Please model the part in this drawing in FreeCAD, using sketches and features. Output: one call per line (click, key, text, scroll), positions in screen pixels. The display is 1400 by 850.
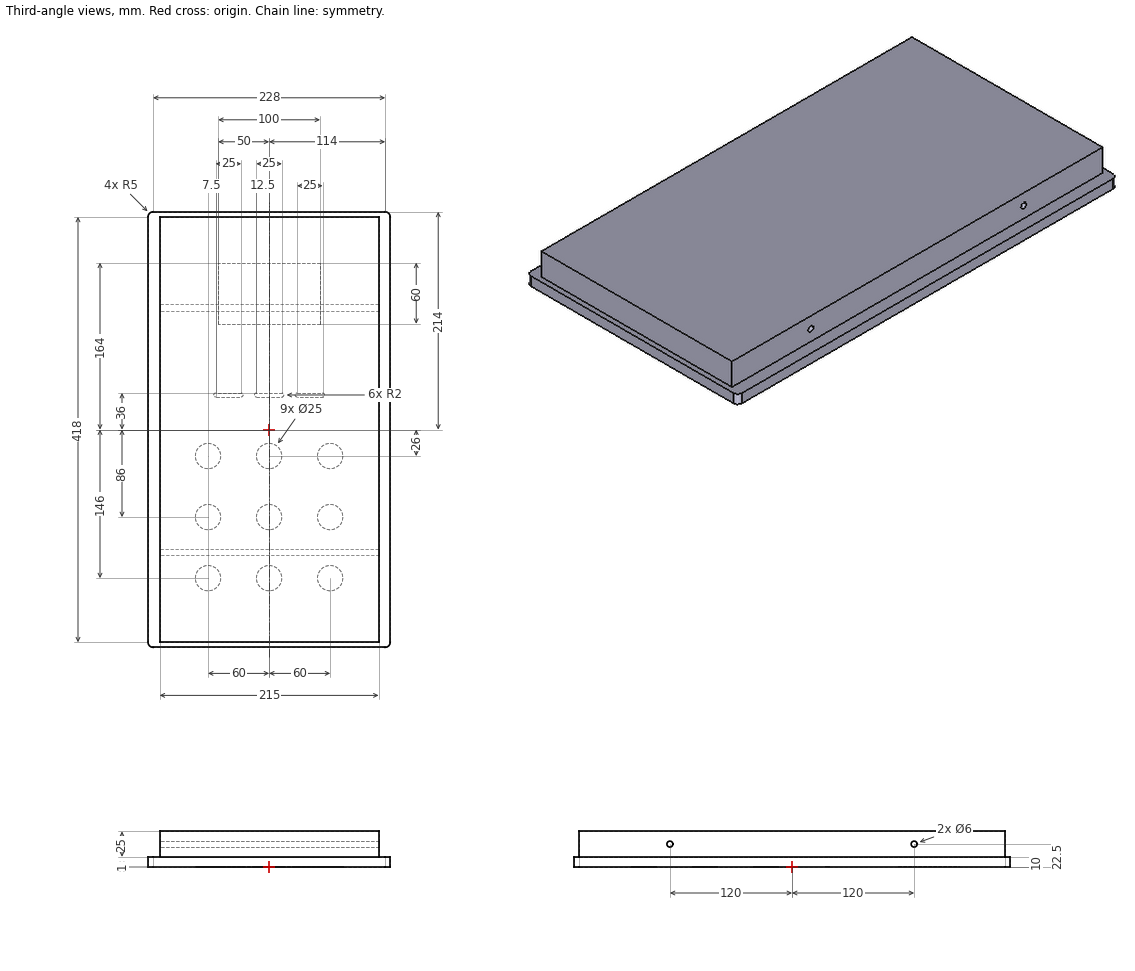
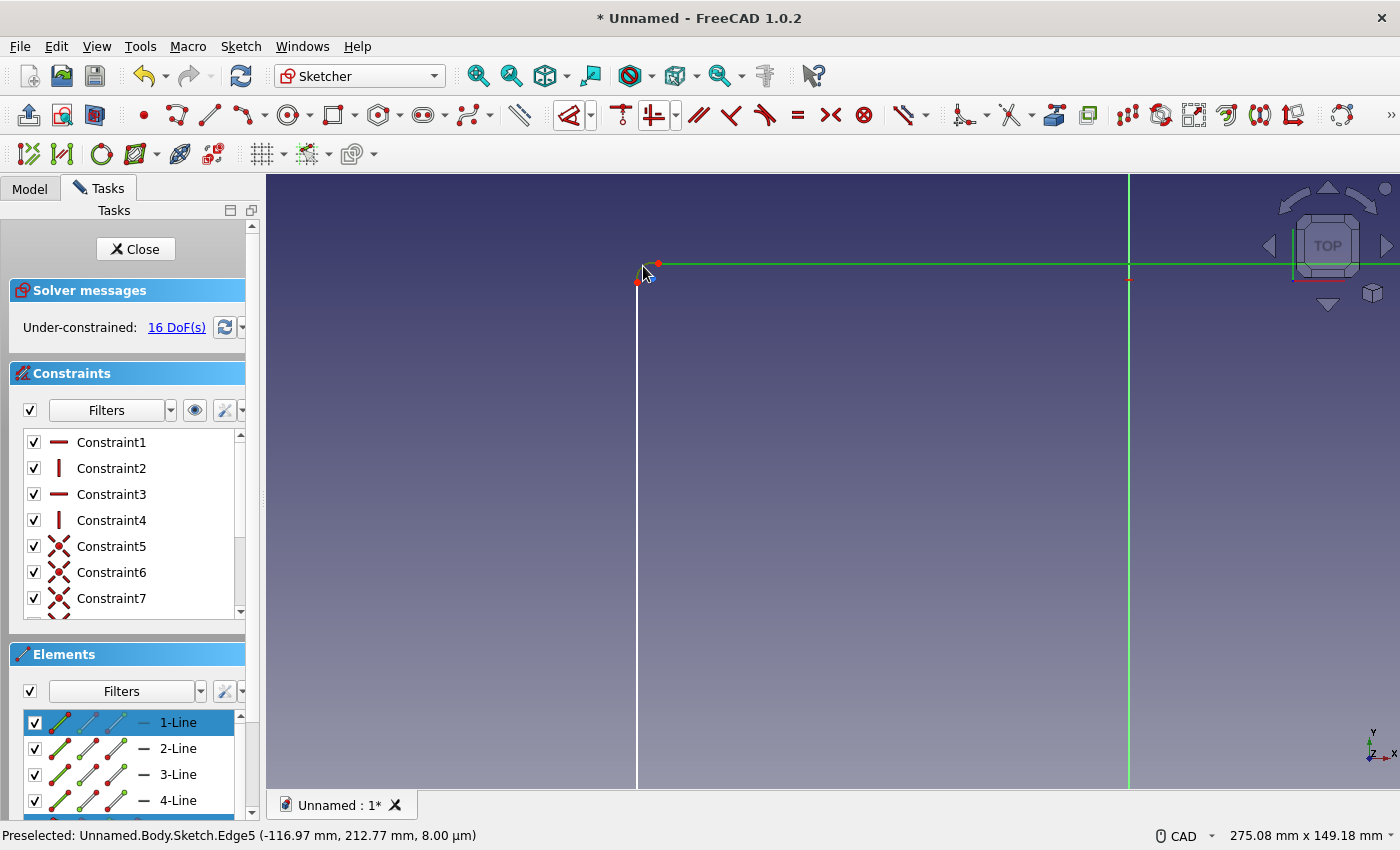
key(t)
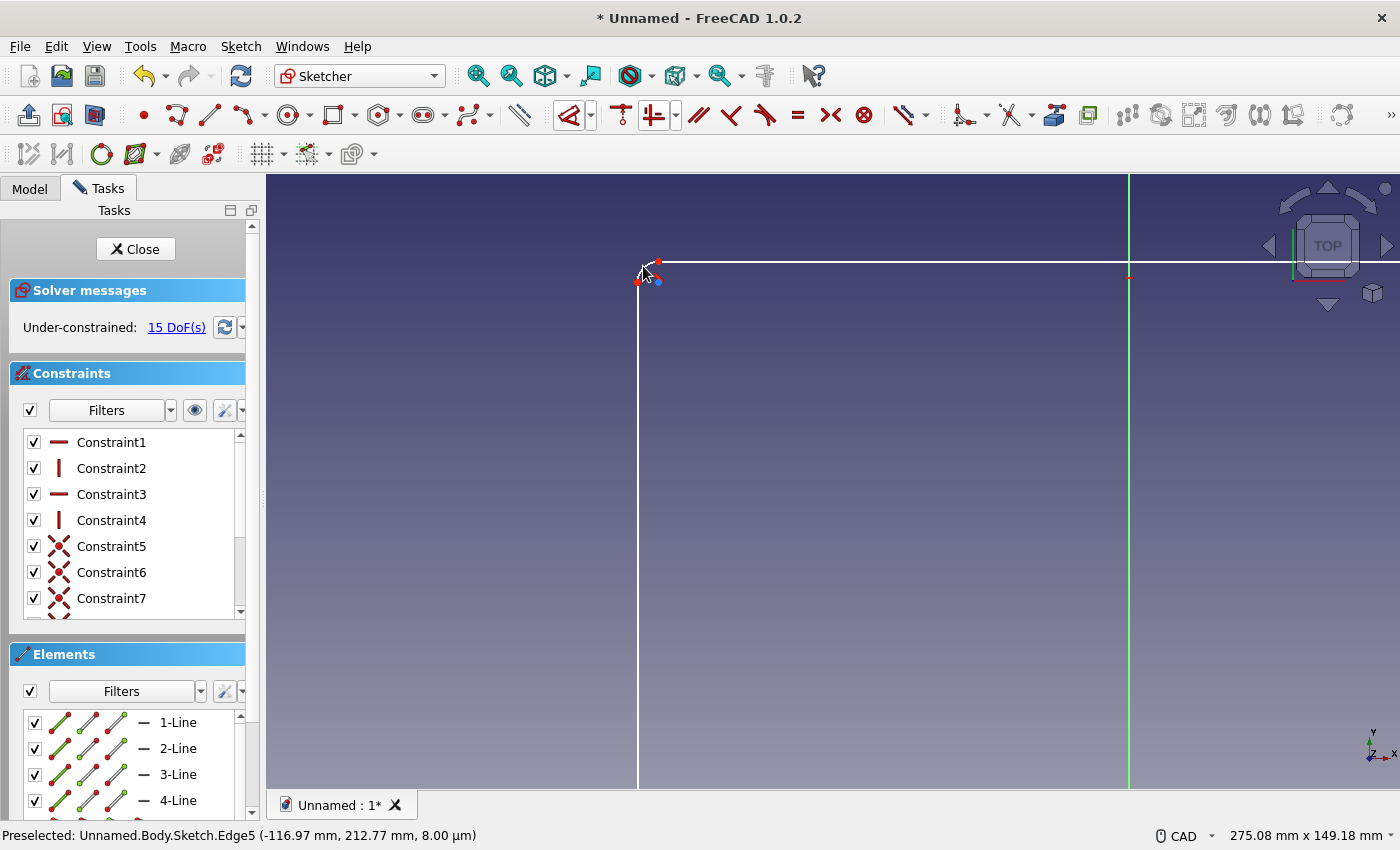
scroll(645, 266, down, 7)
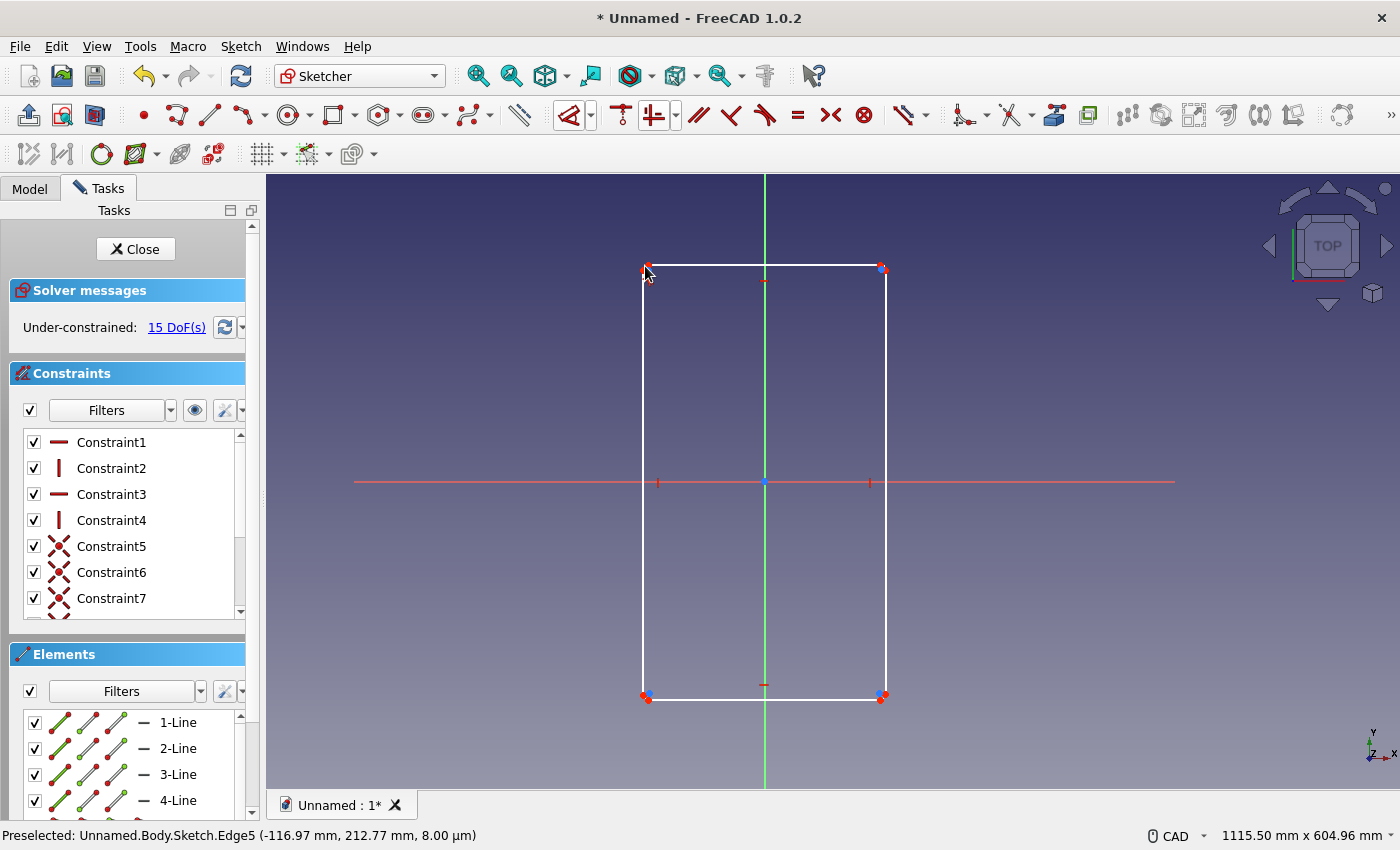
click(718, 265)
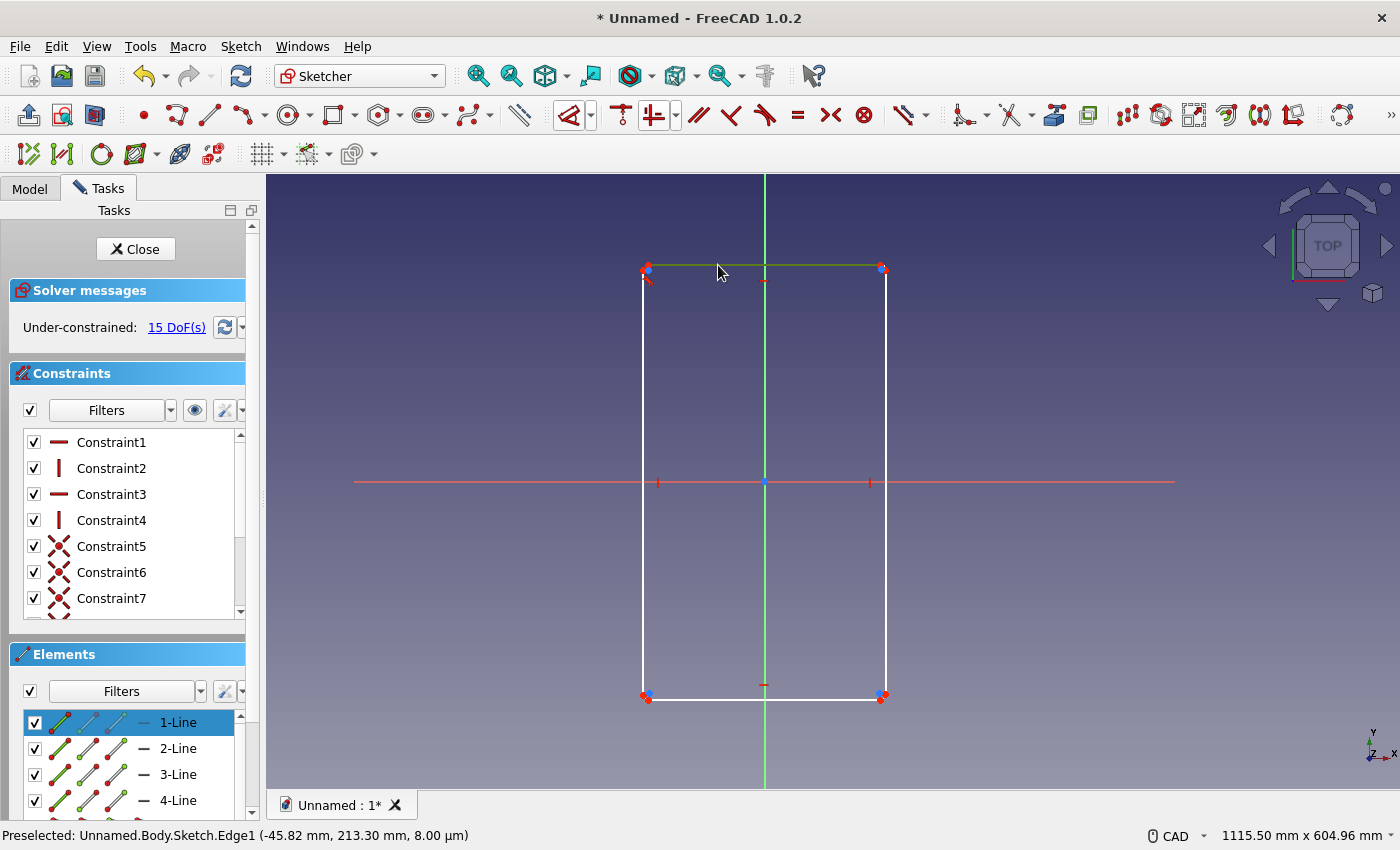
scroll(885, 266, up, 7)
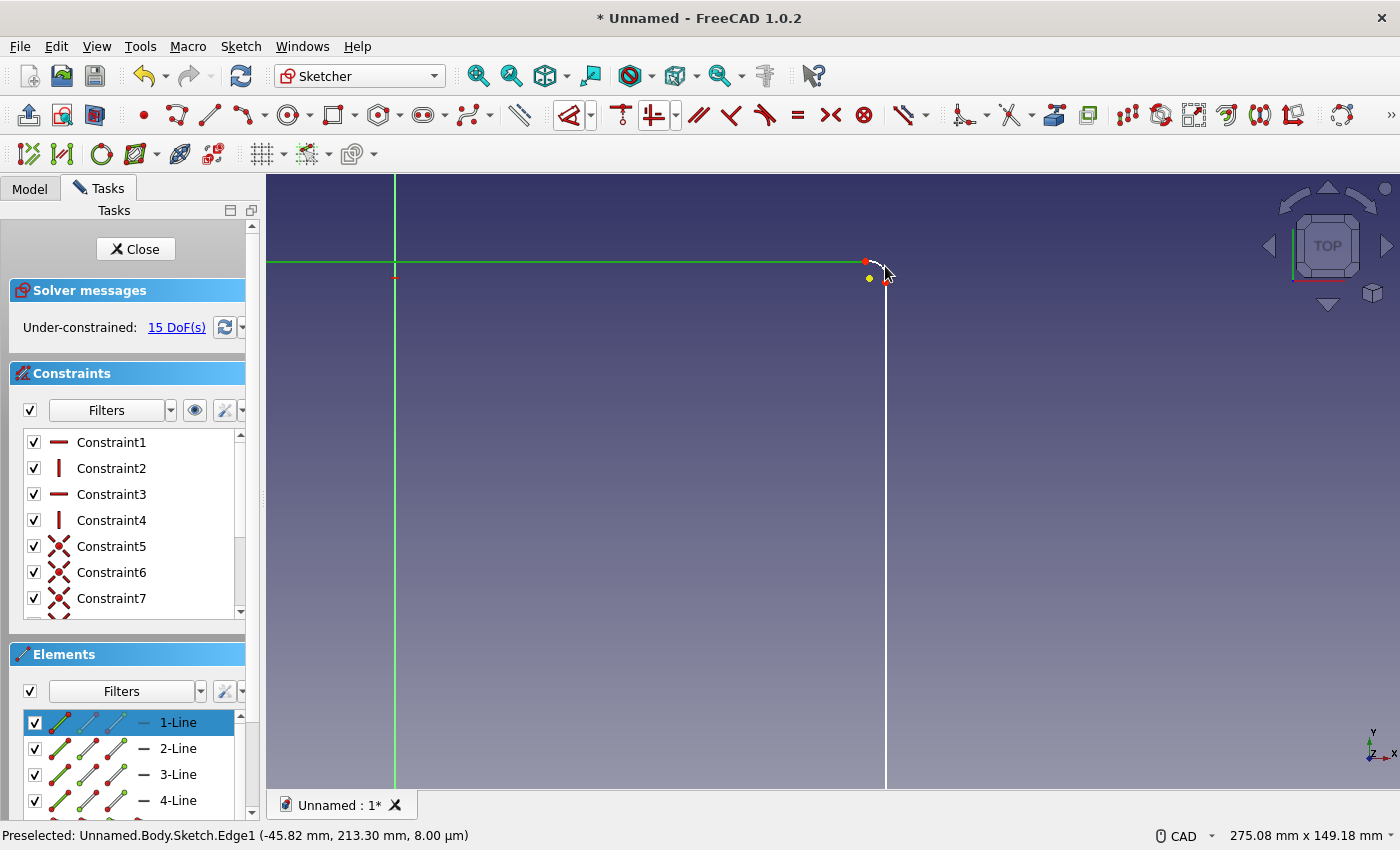
click(882, 266)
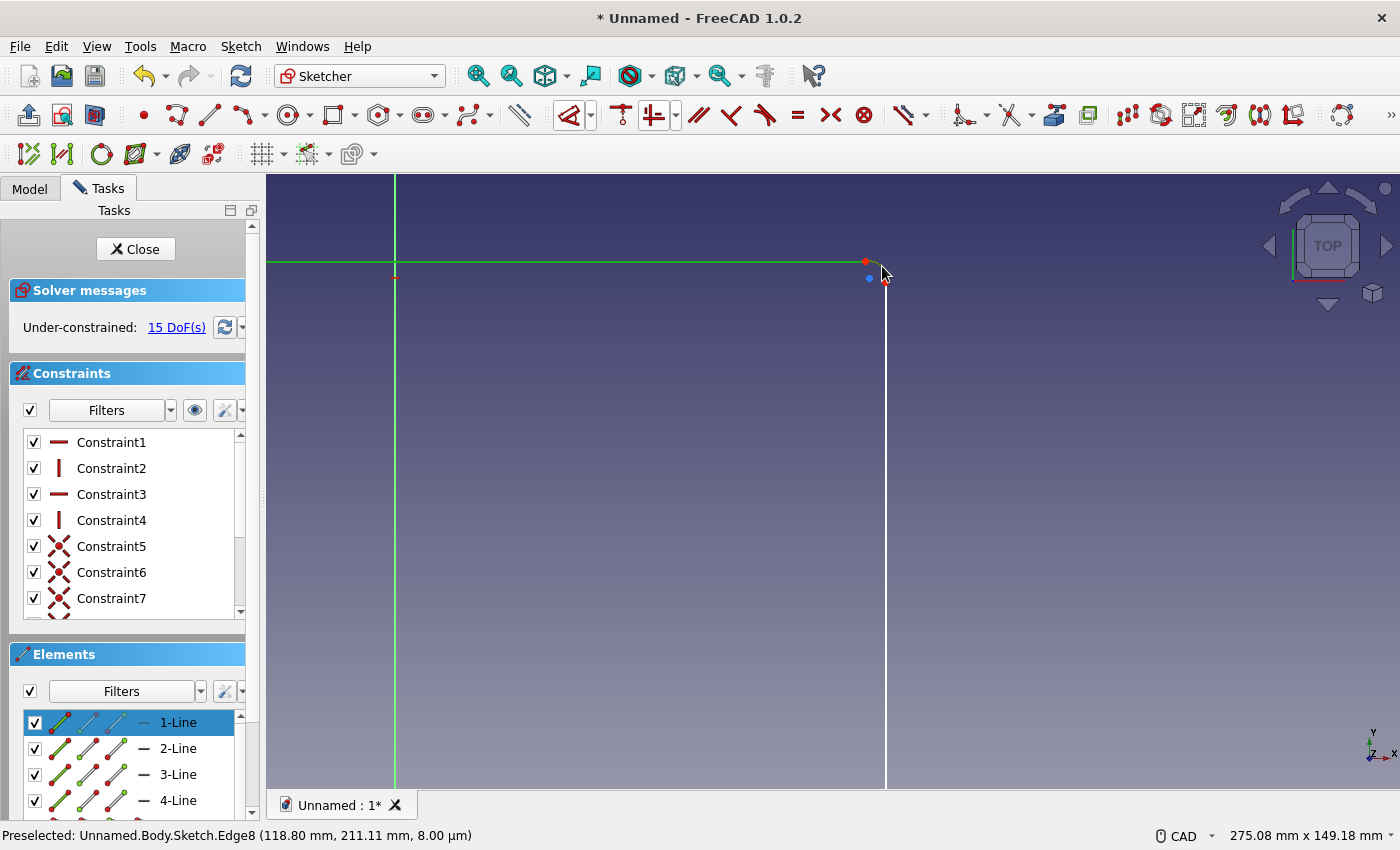
key(t)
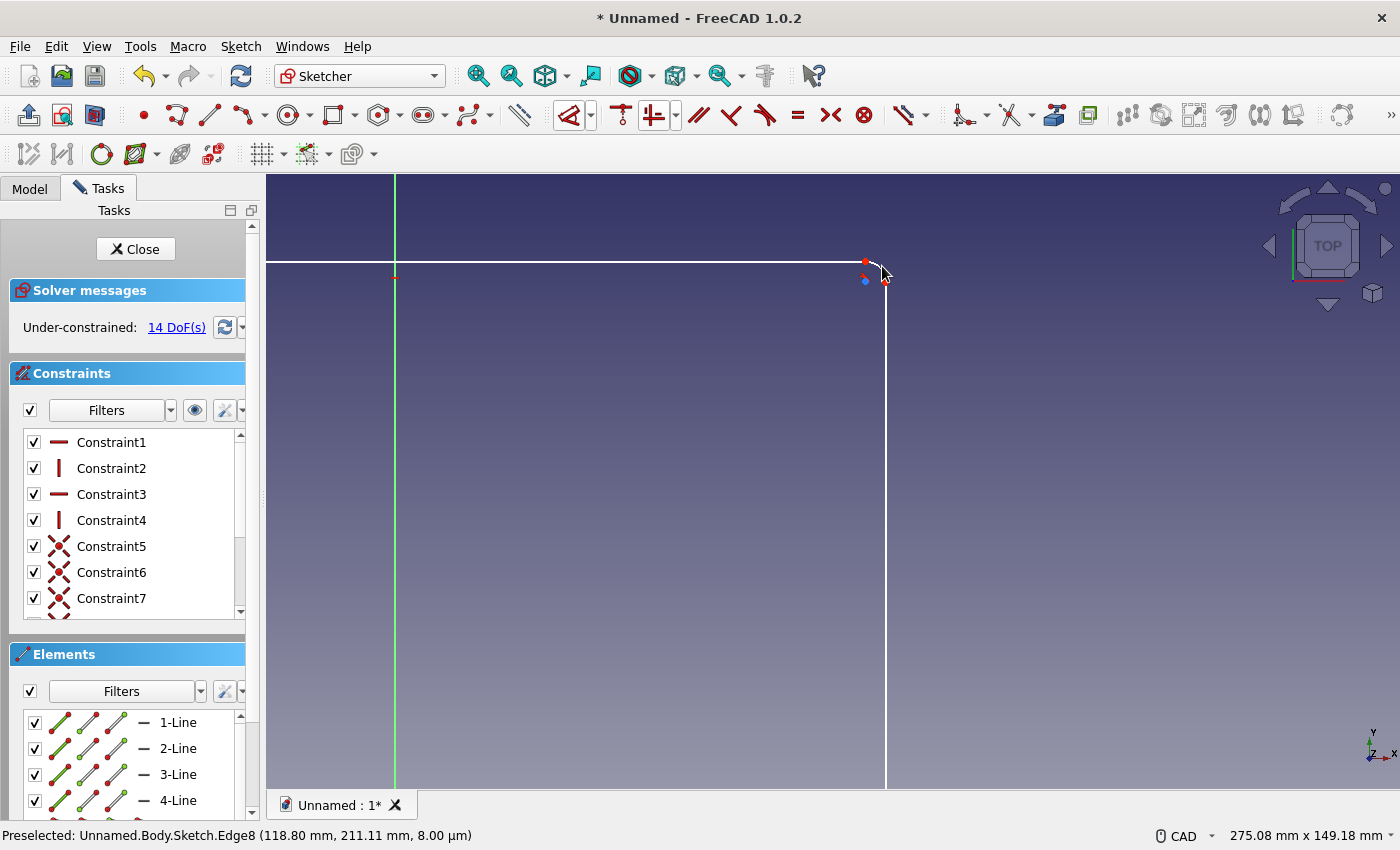
scroll(885, 266, down, 7)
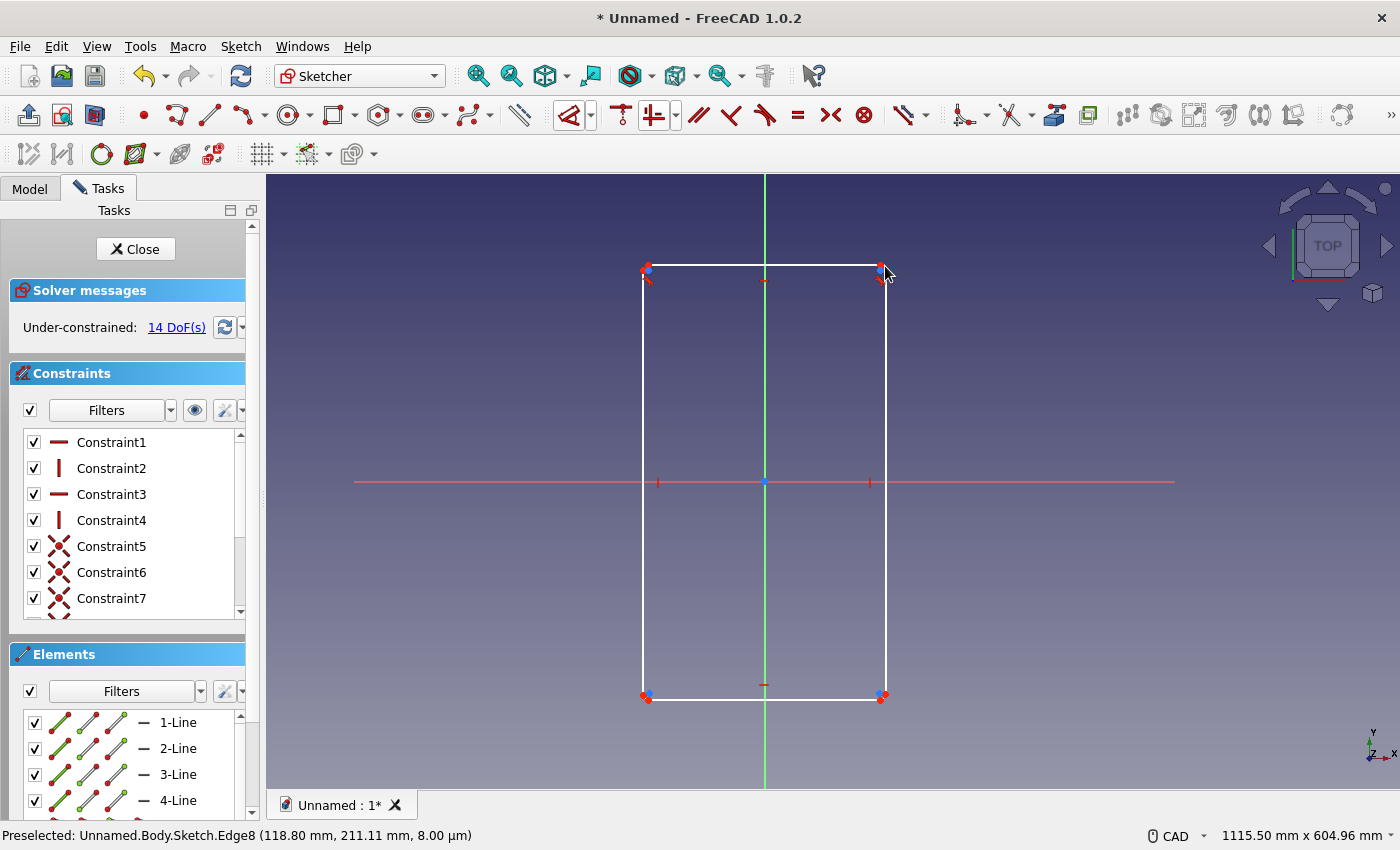
click(643, 398)